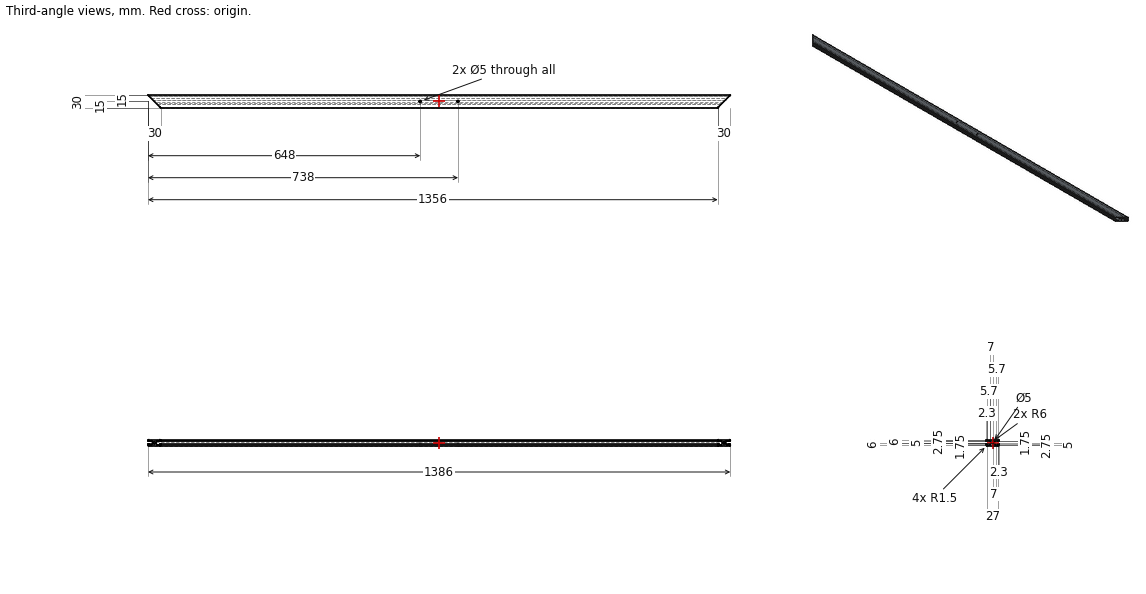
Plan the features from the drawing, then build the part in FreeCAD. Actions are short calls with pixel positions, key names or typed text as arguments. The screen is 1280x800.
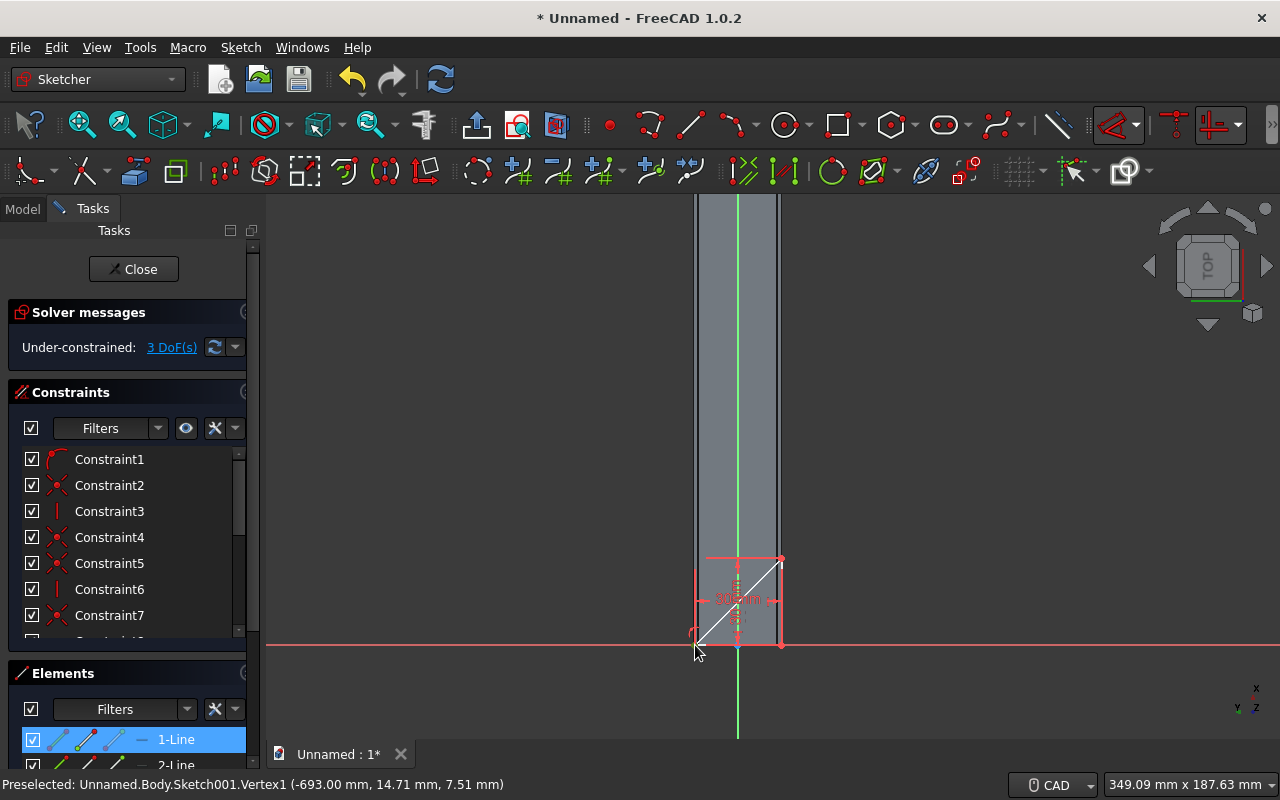
key(l)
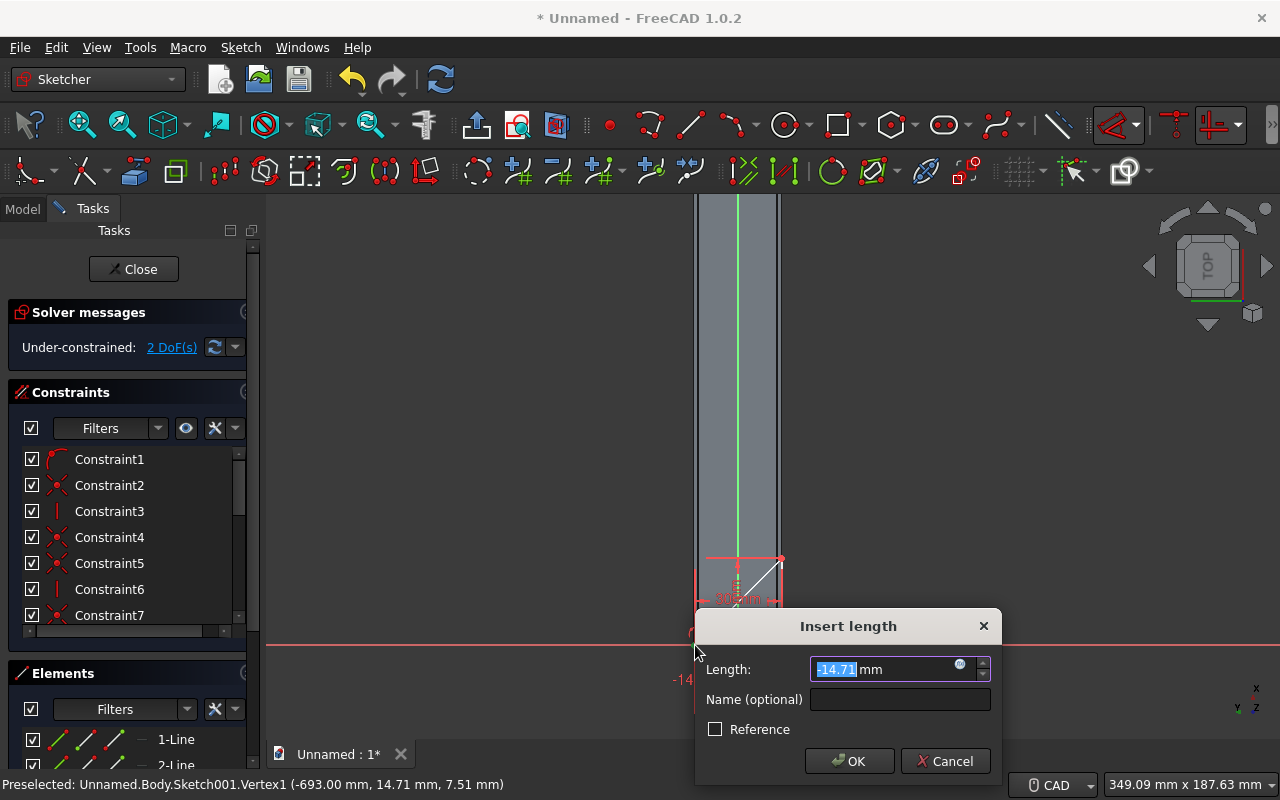
text(-15)
key(Return)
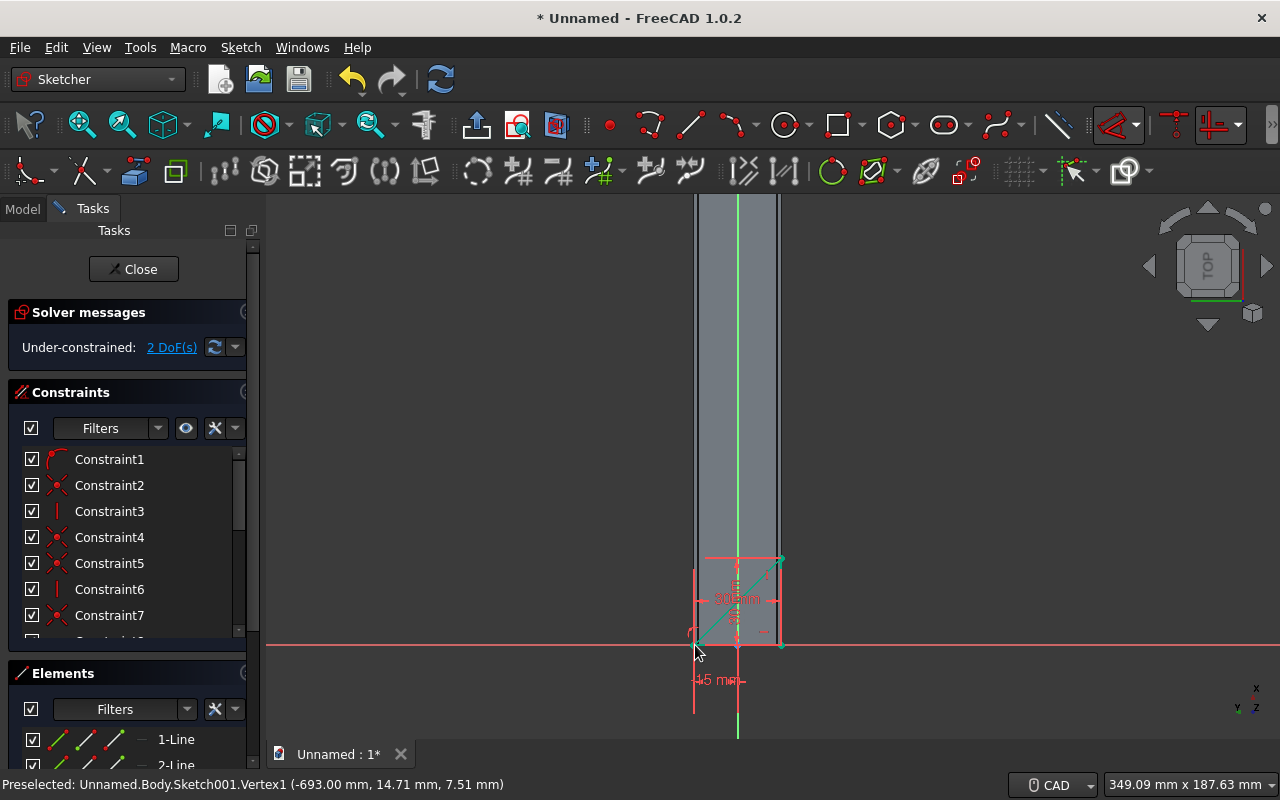
scroll(701, 649, down, 12)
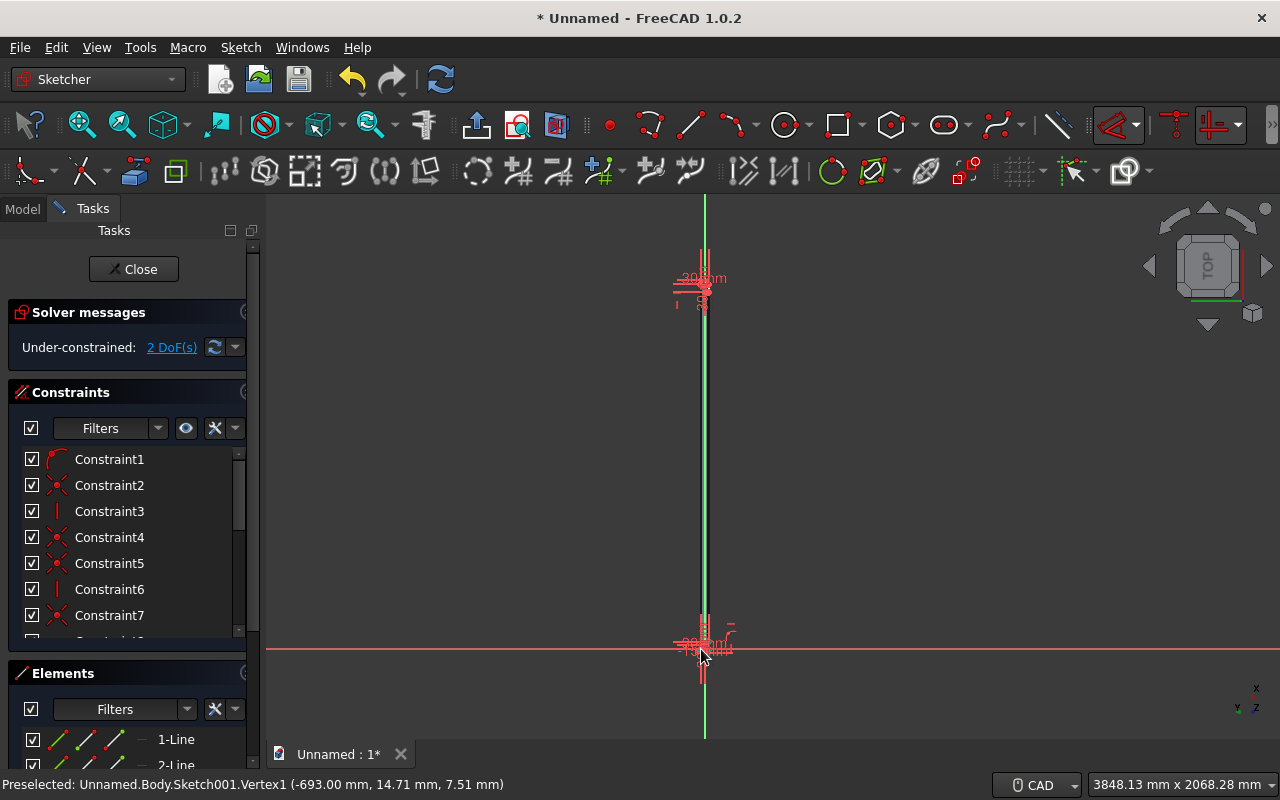
scroll(709, 292, up, 12)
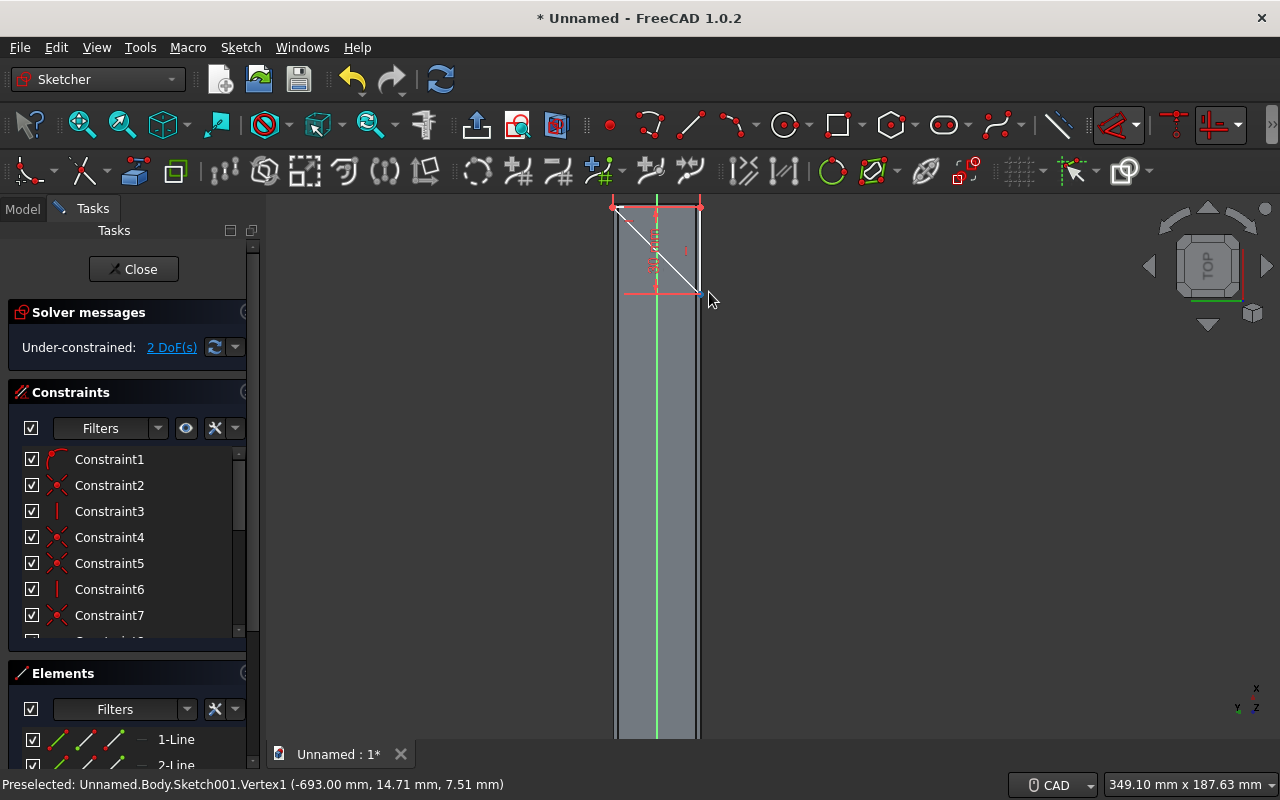
click(700, 294)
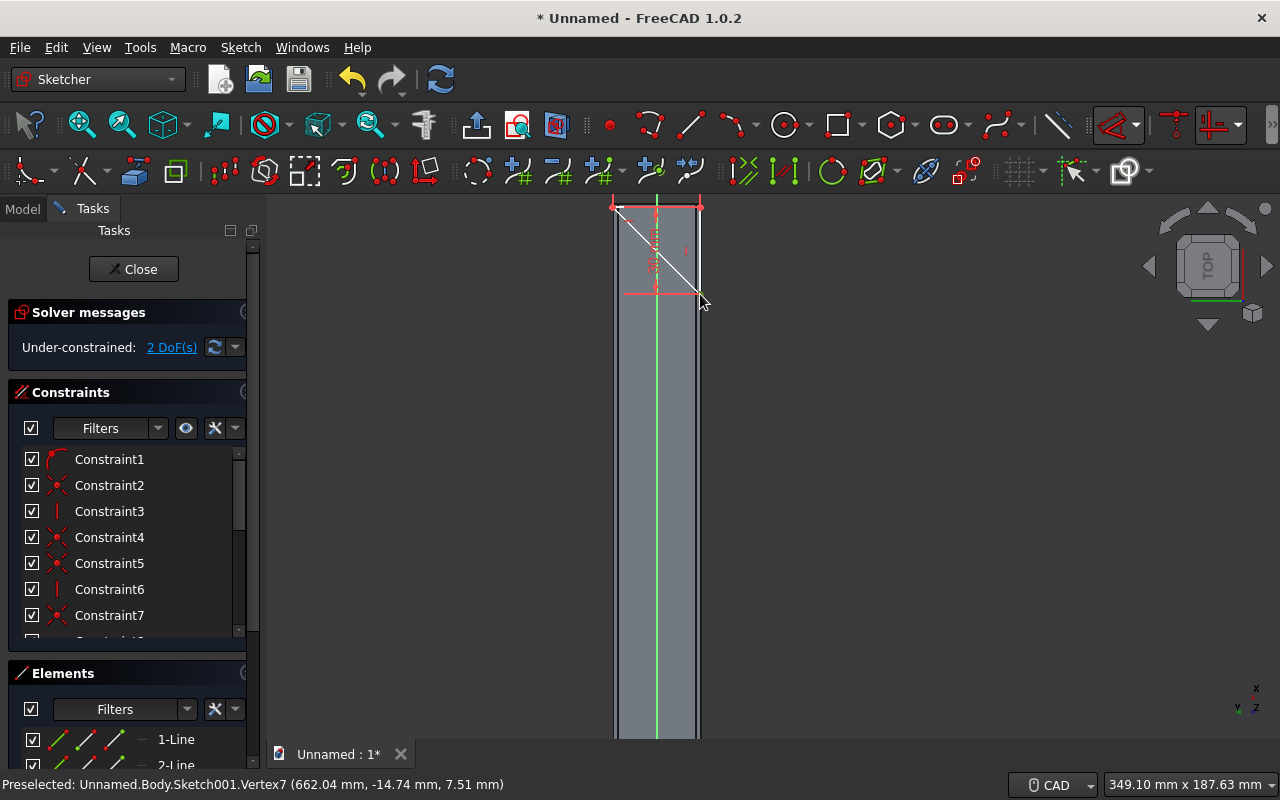
click(1138, 126)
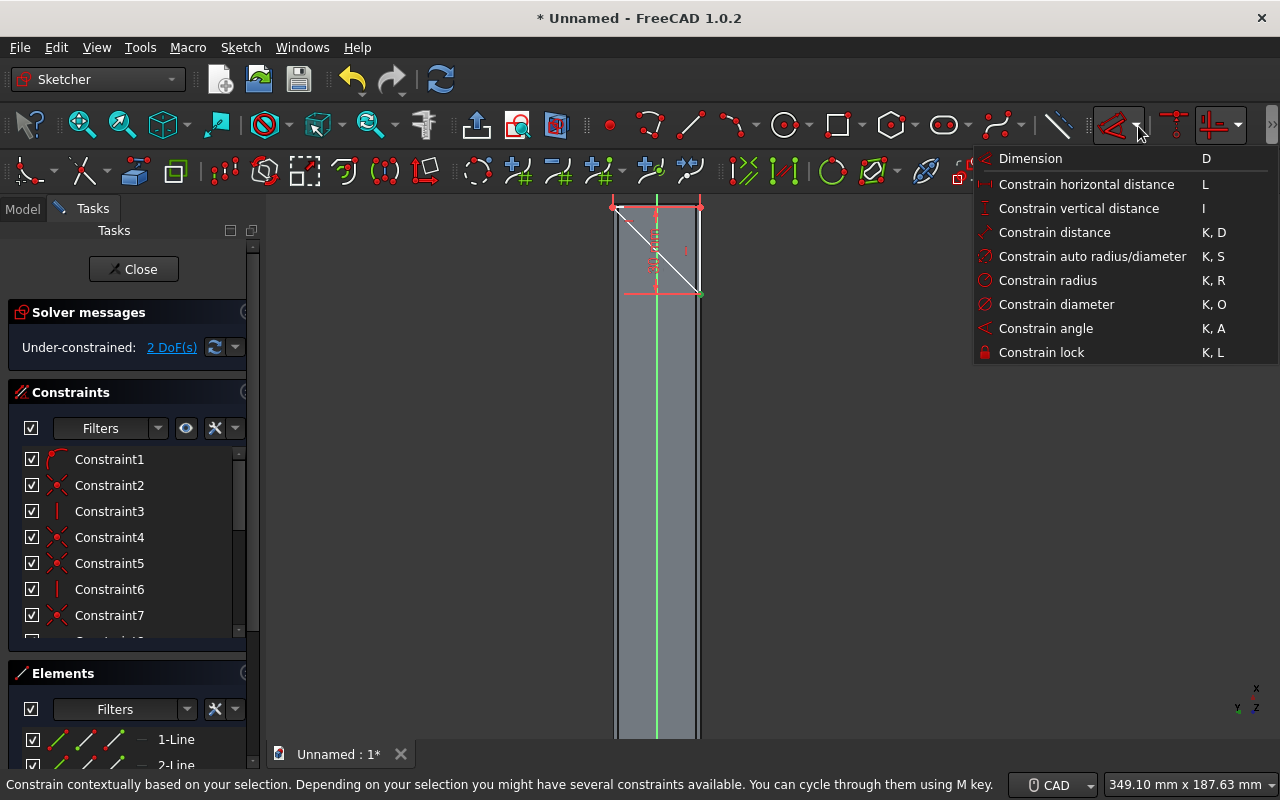
click(1126, 184)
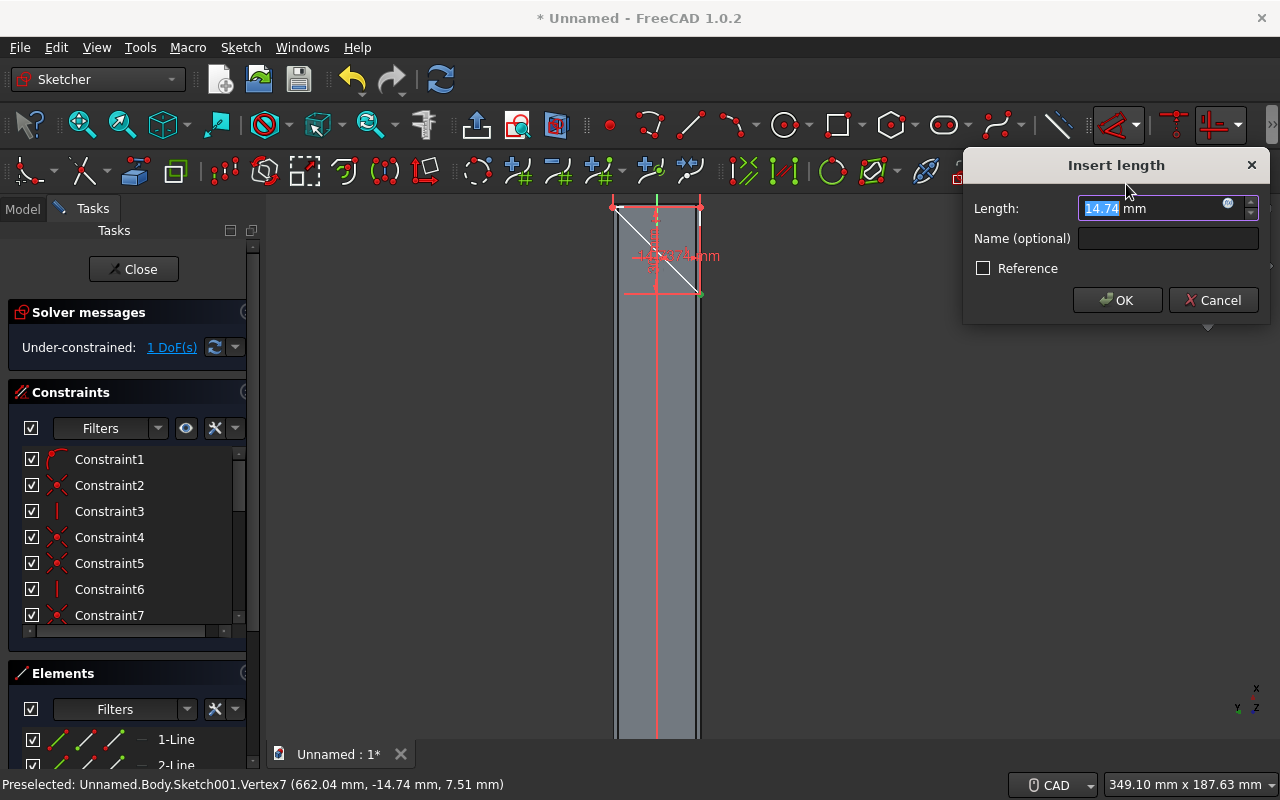
text(15)
key(Return)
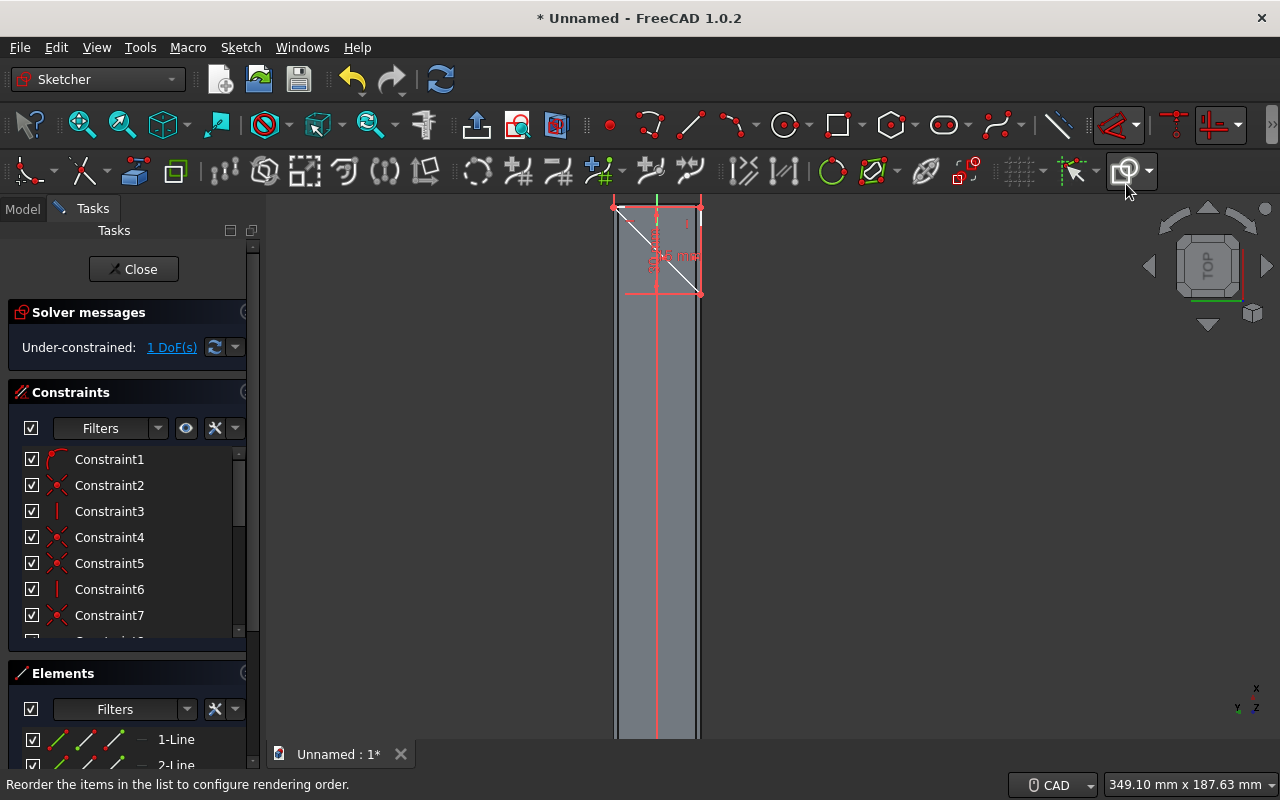
scroll(709, 292, down, 12)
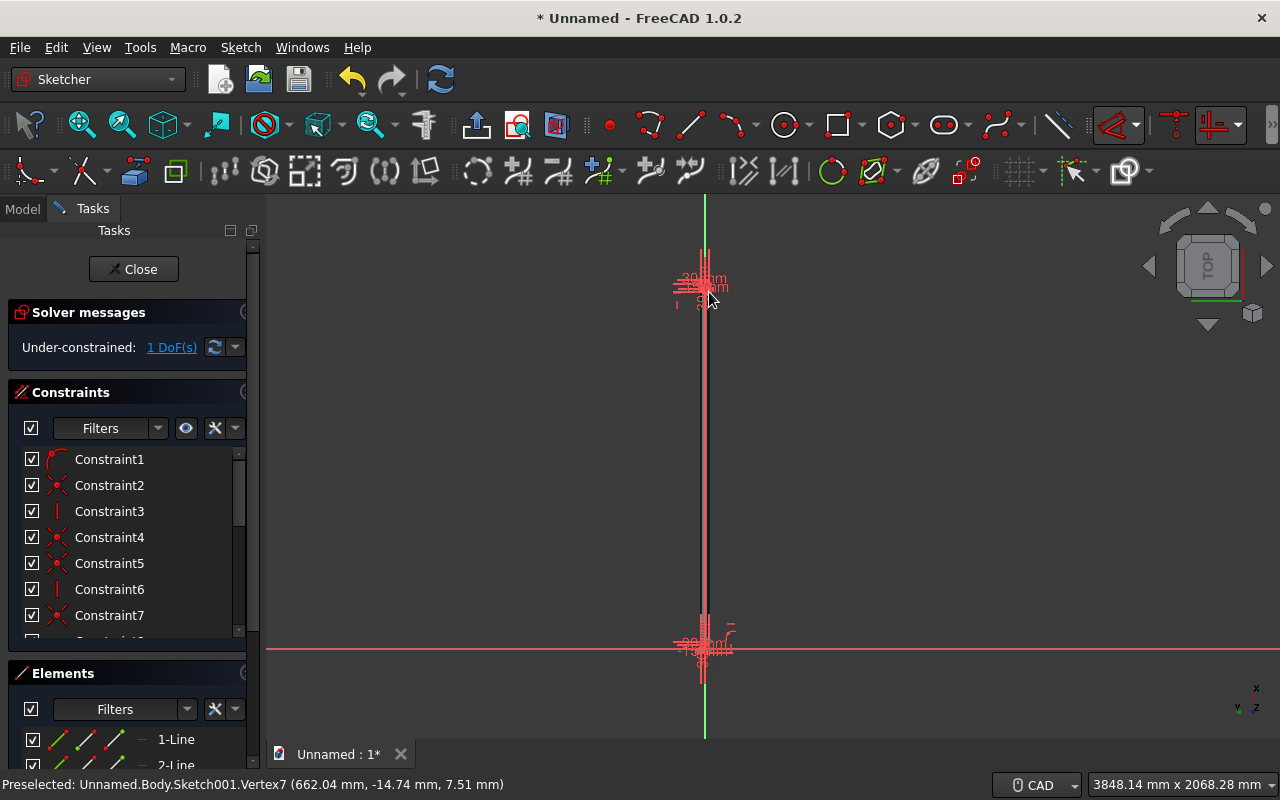
scroll(709, 292, up, 3)